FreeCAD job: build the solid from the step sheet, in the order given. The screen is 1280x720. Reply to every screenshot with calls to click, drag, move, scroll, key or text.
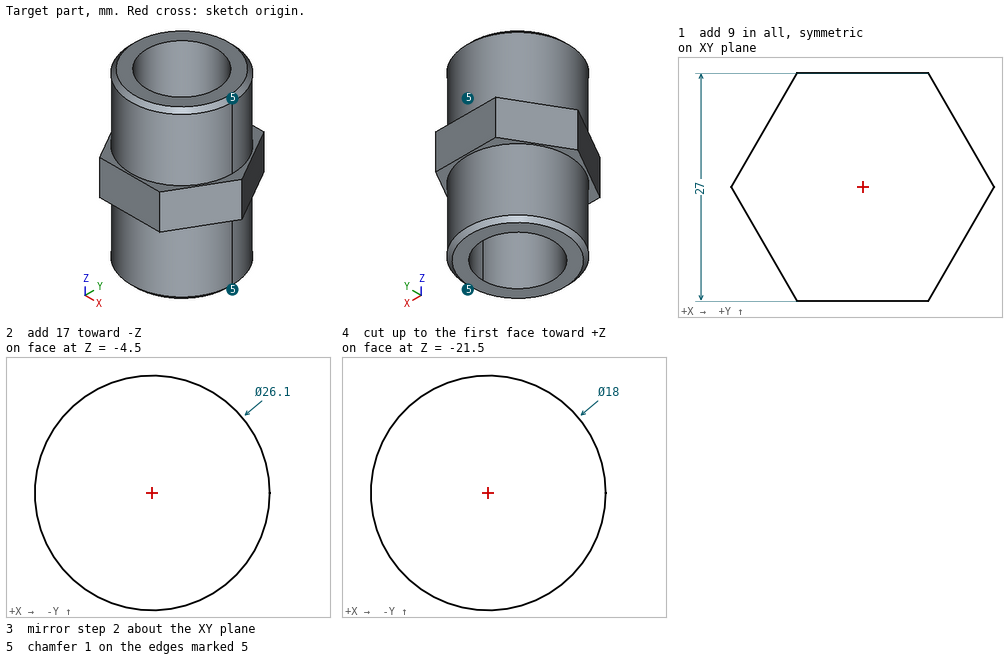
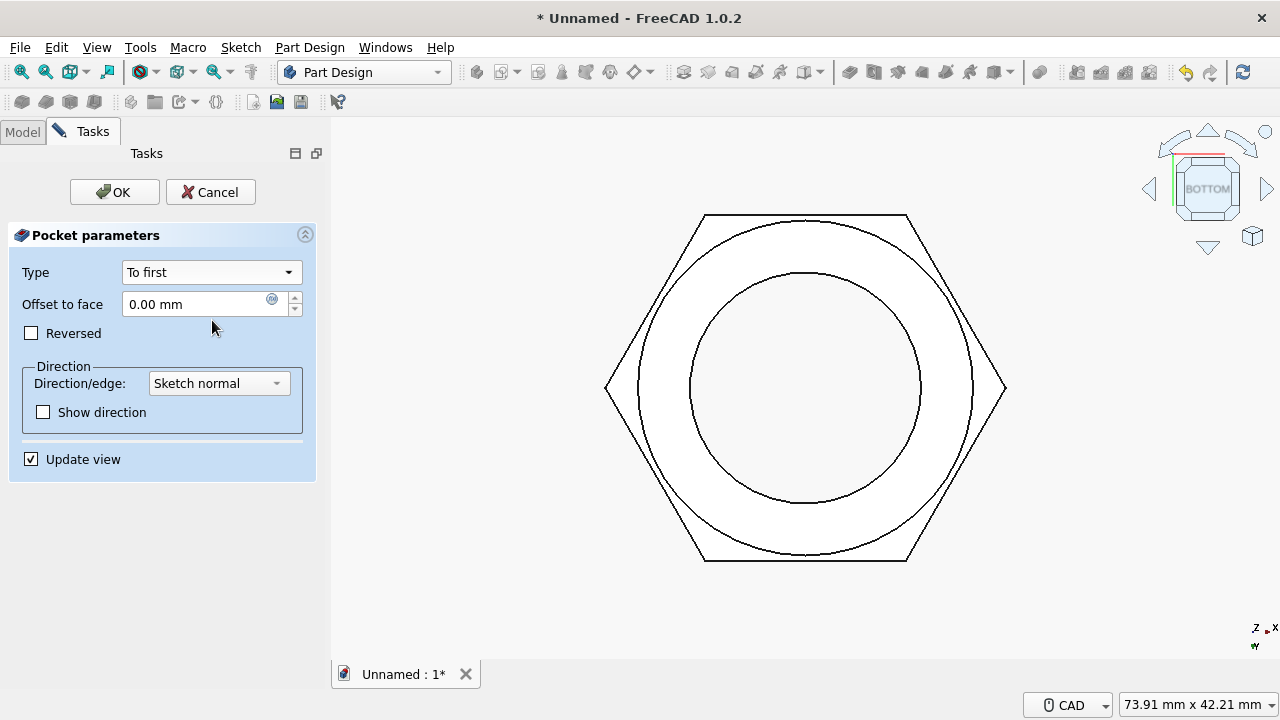
click(115, 192)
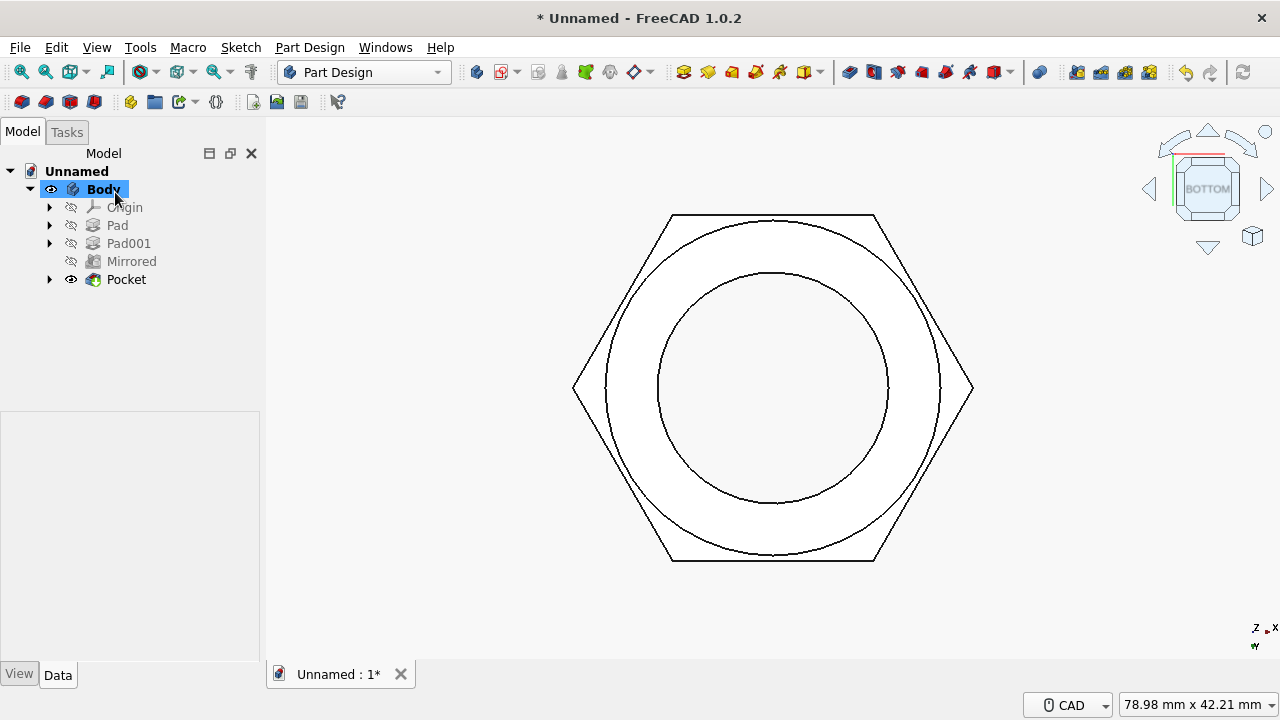
click(605, 387)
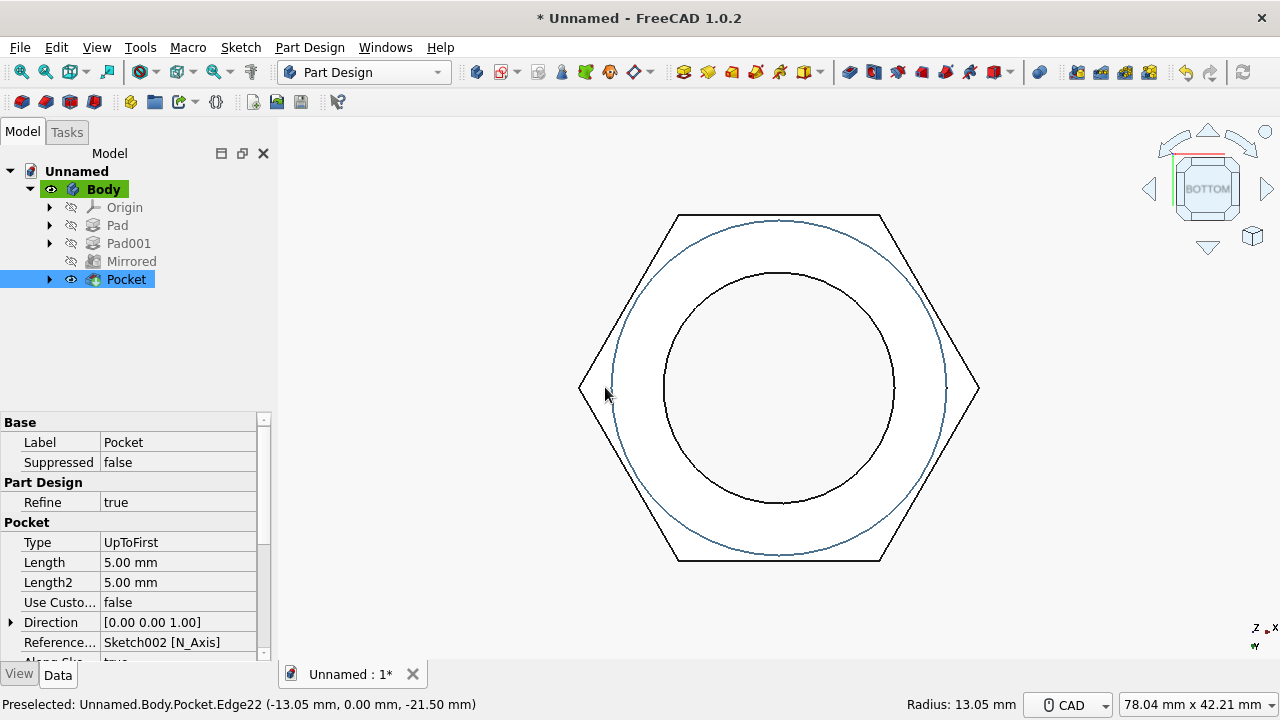
key(0)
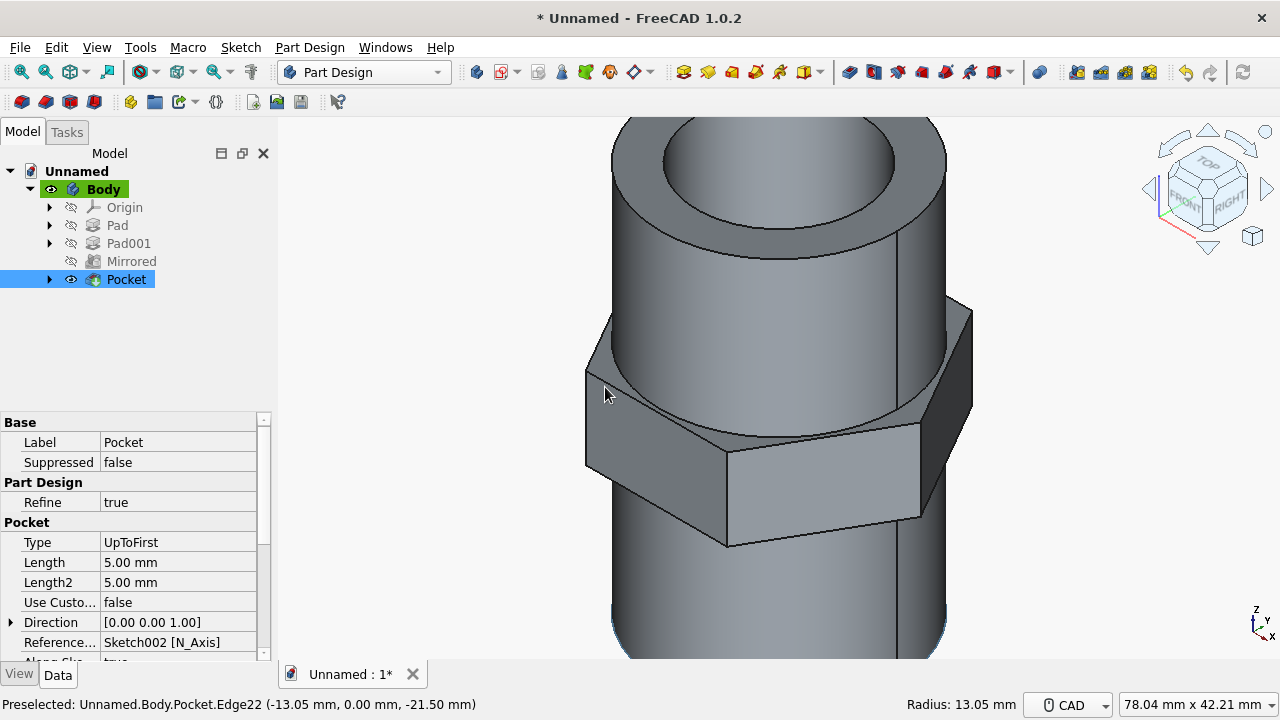
key(v)
key(f)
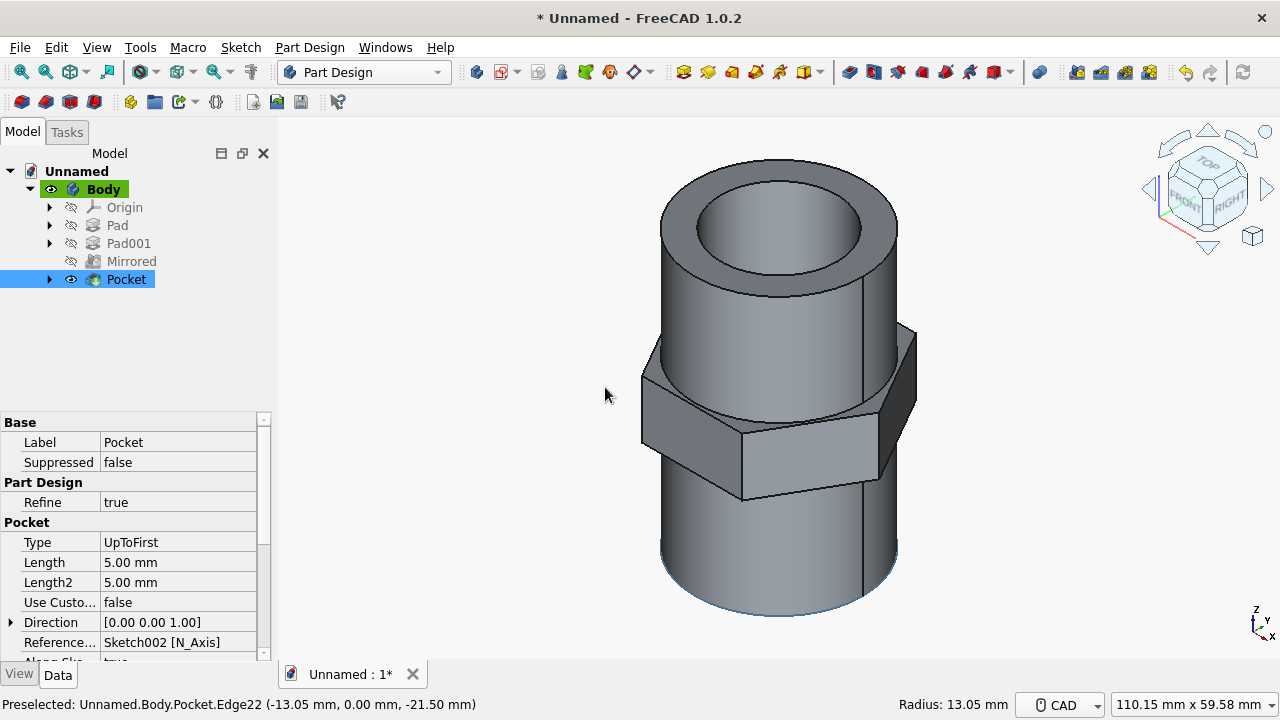
click(673, 258, ctrl)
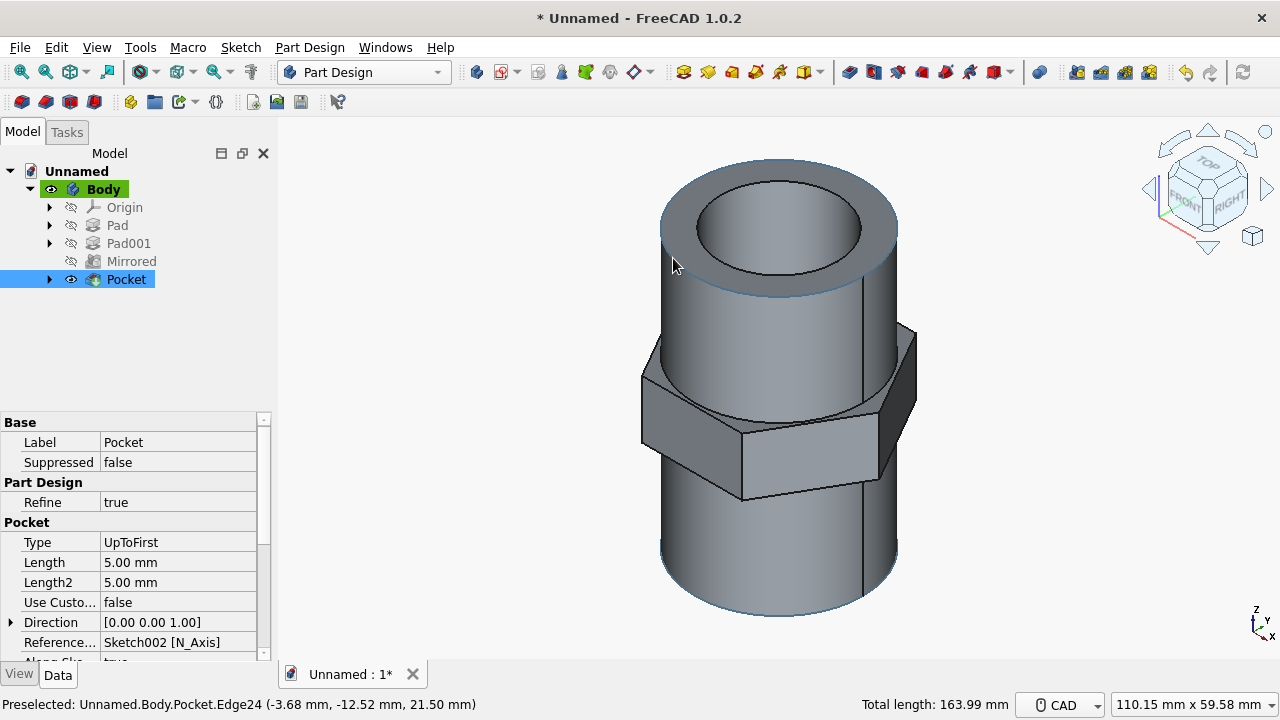
click(46, 102)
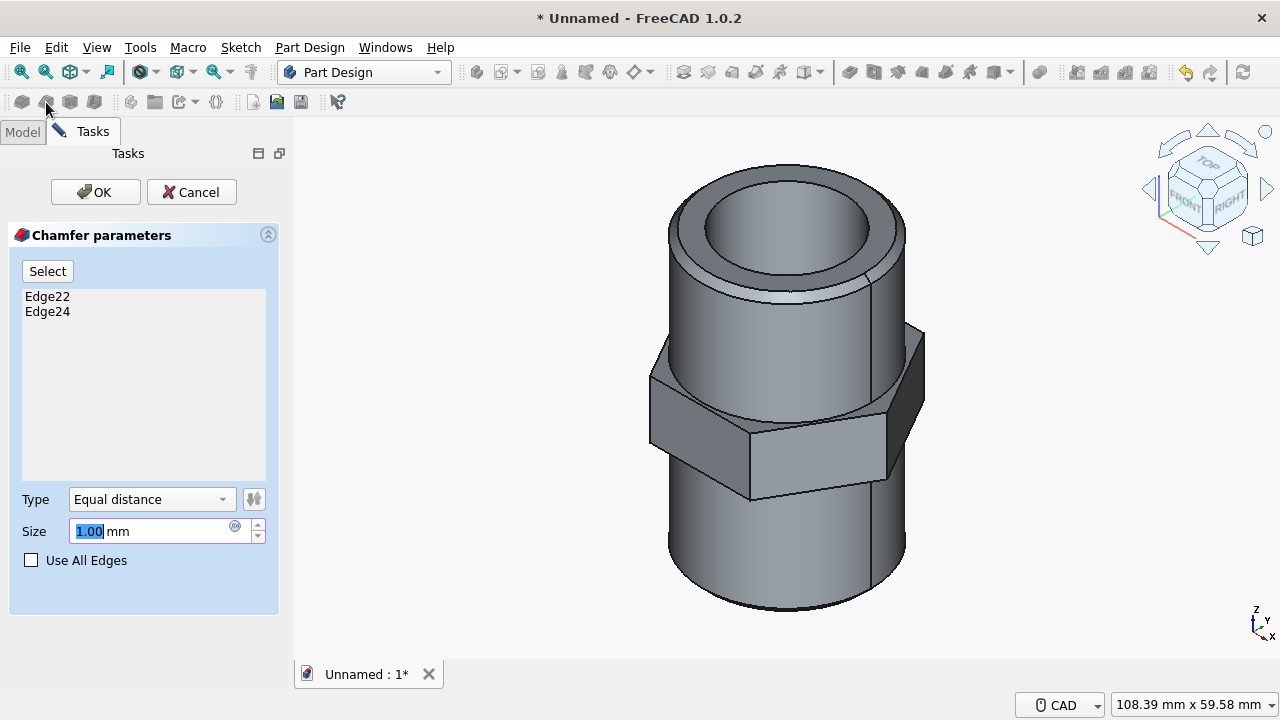
text(1)
key(Tab)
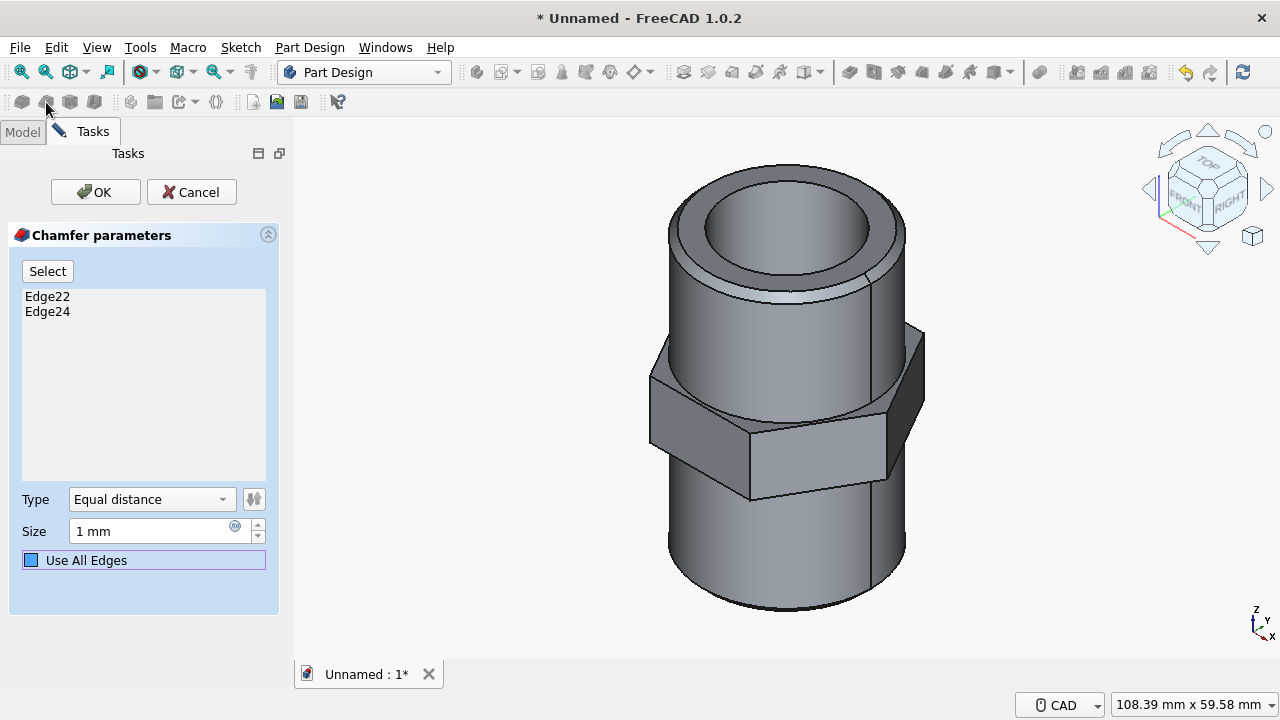
click(96, 192)